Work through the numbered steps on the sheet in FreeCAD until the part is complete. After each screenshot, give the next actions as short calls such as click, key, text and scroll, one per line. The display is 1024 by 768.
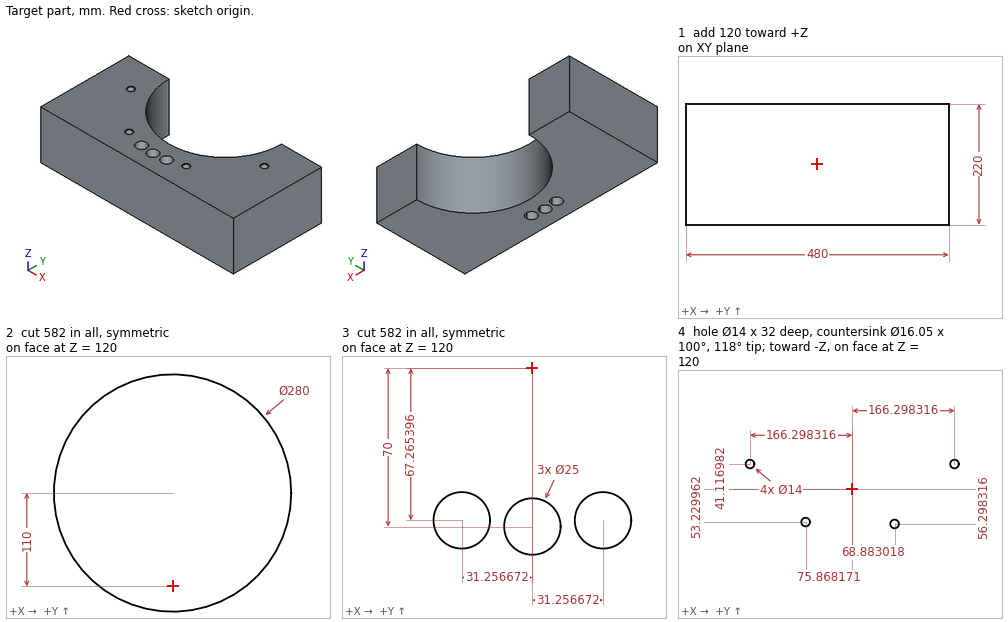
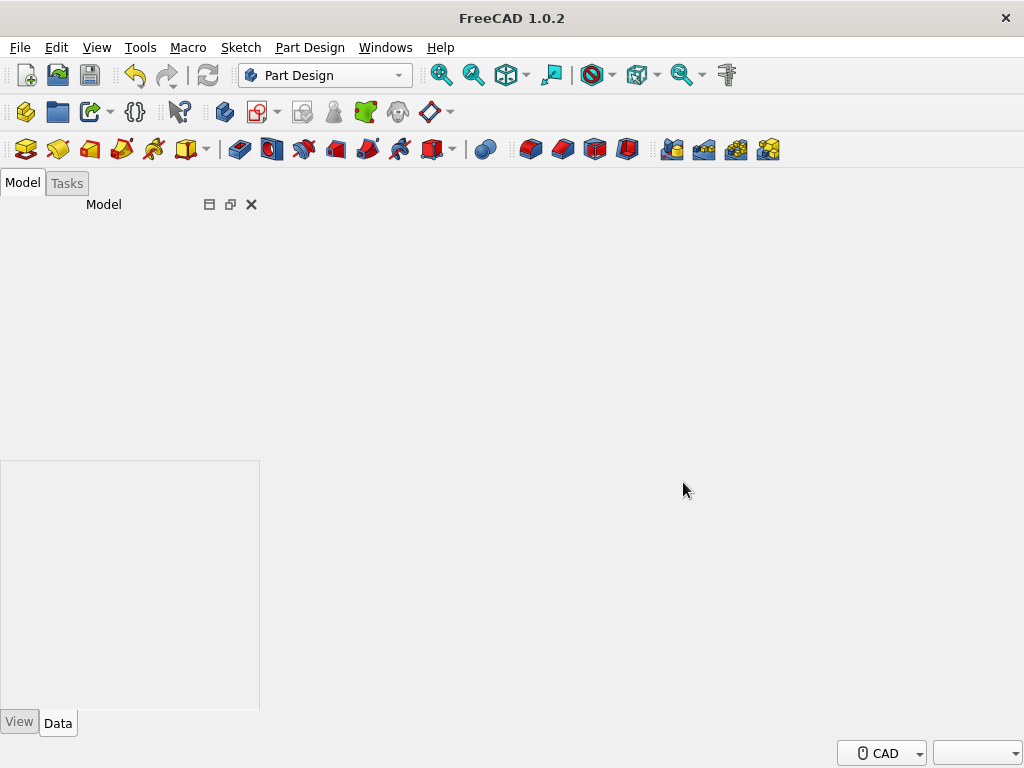
key(ctrl+n)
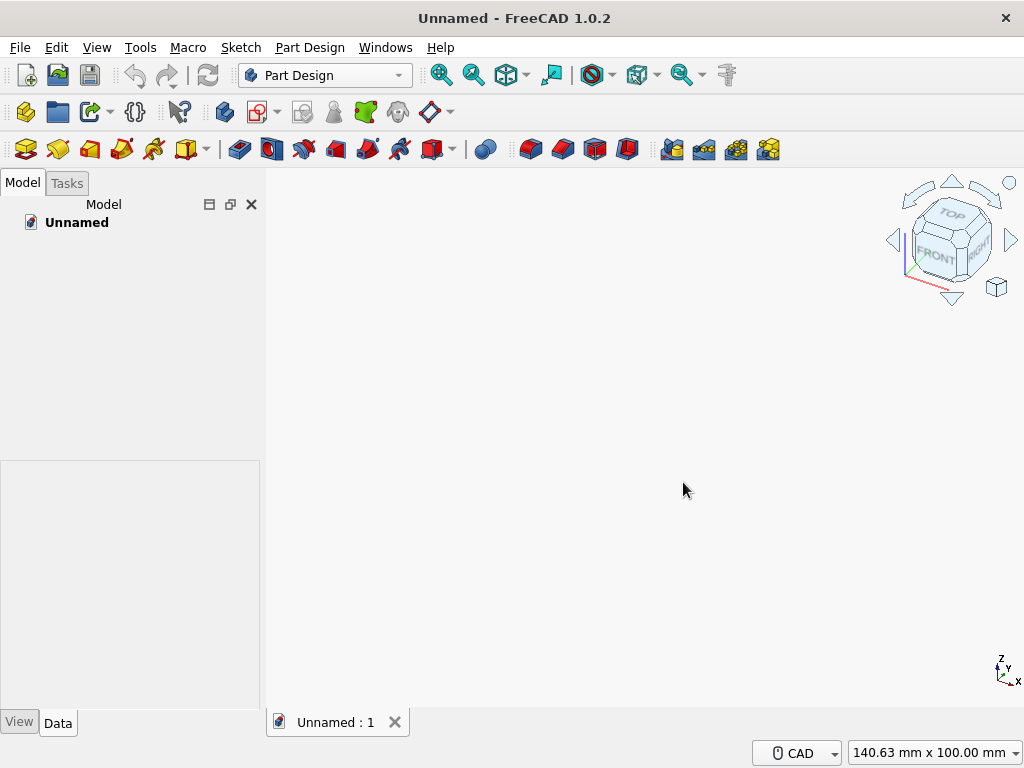
click(258, 112)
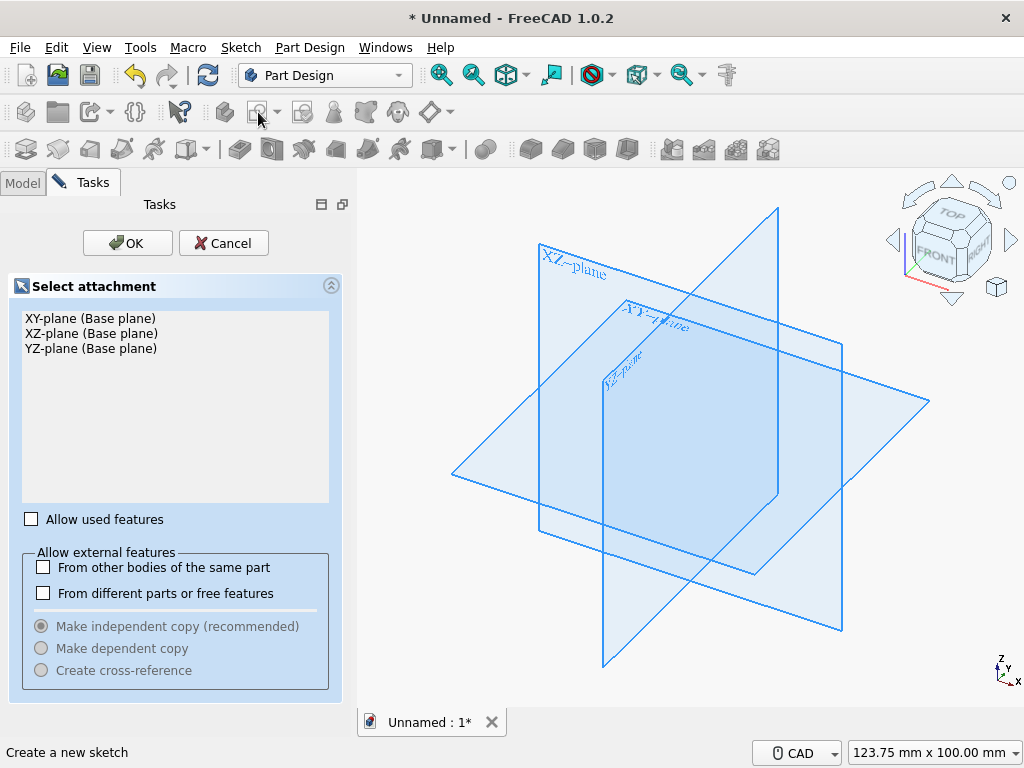
click(82, 318)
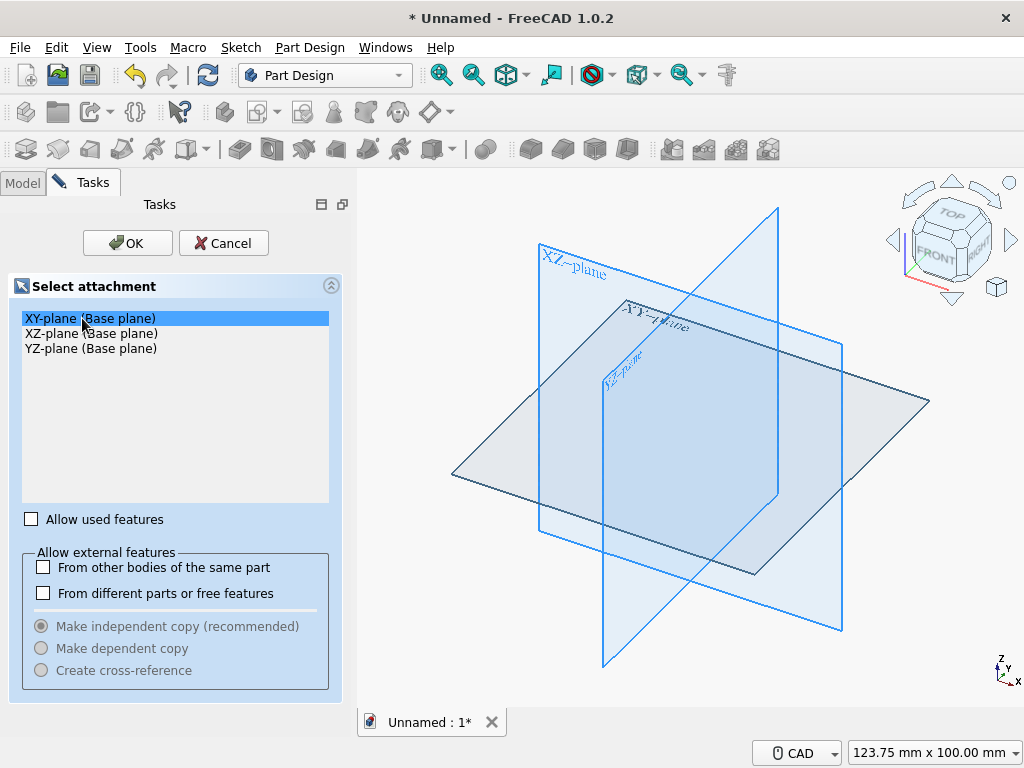
click(128, 243)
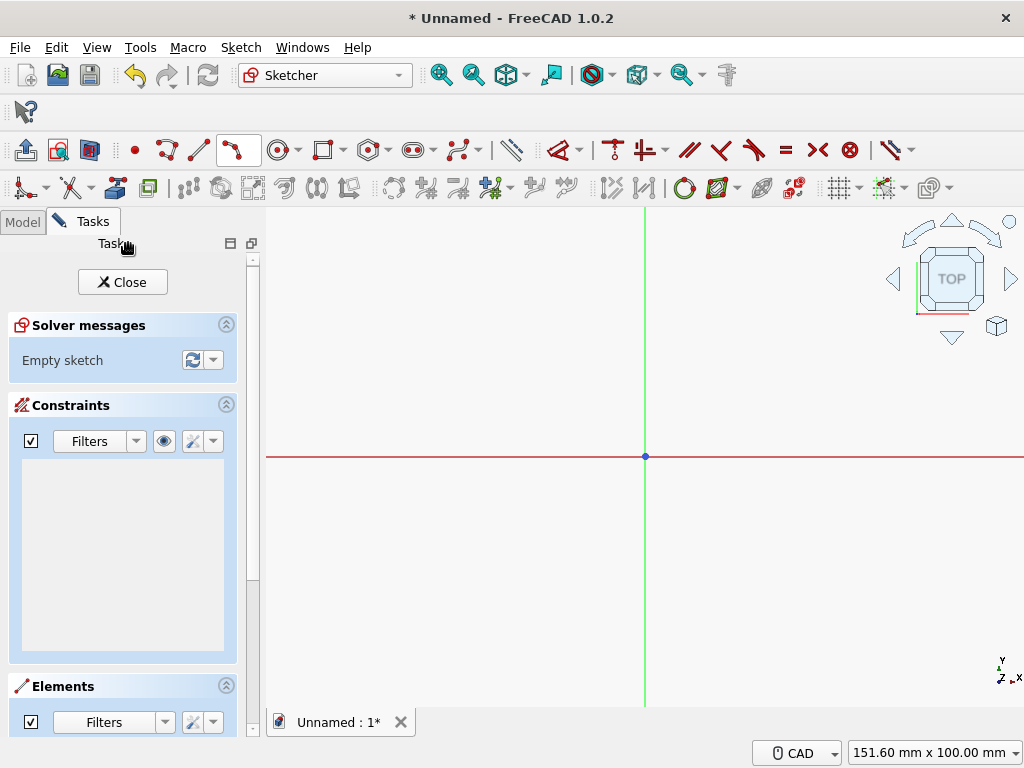
scroll(563, 457, down, 9)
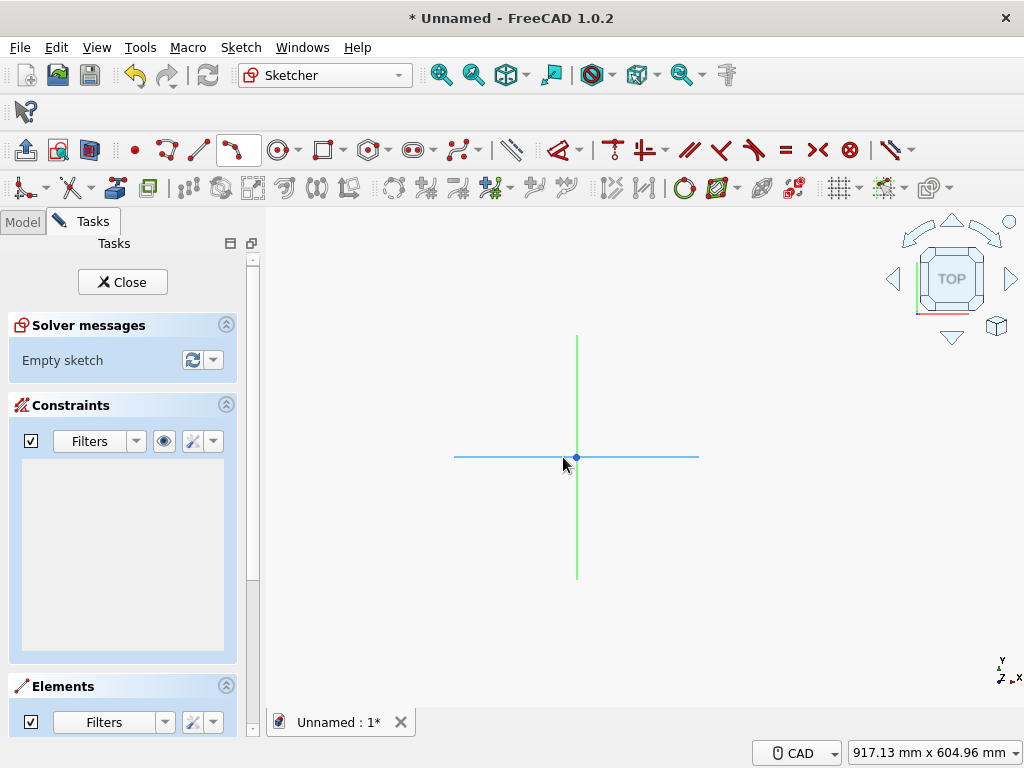
click(346, 150)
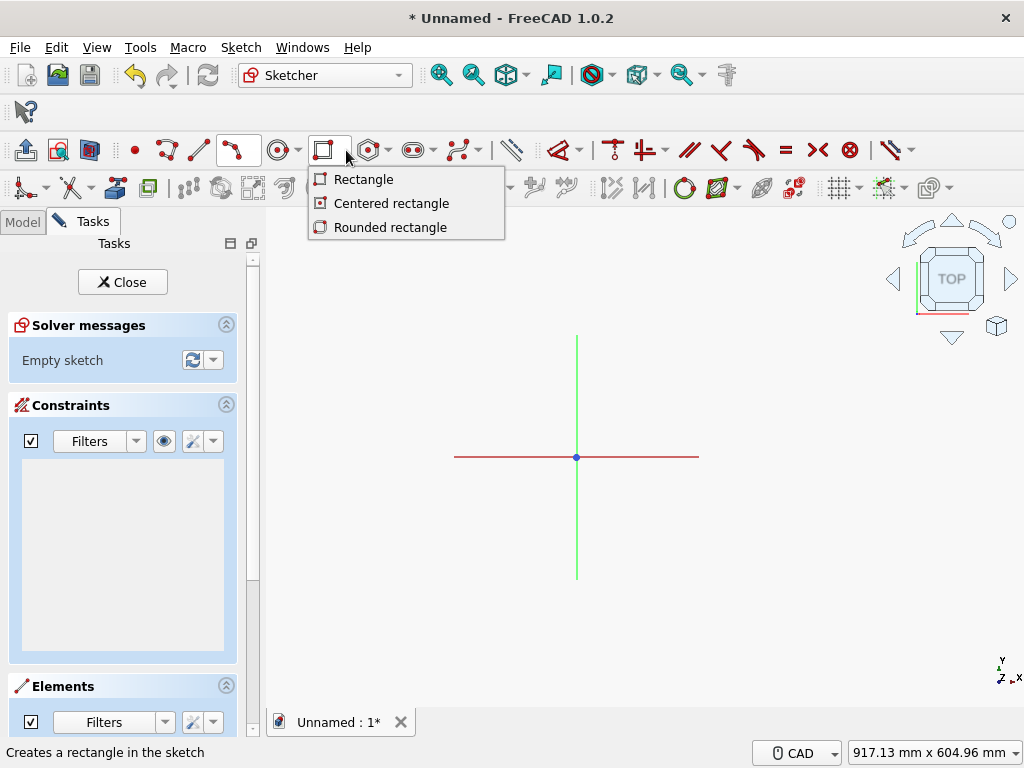
click(406, 203)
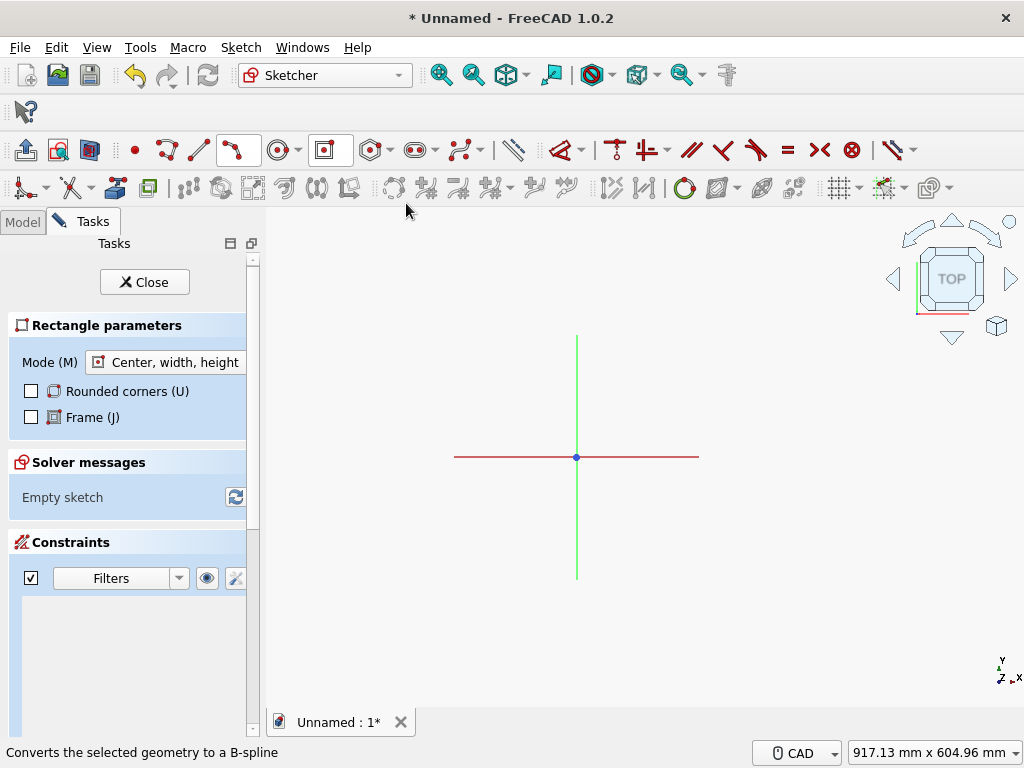
click(577, 457)
move(775, 367)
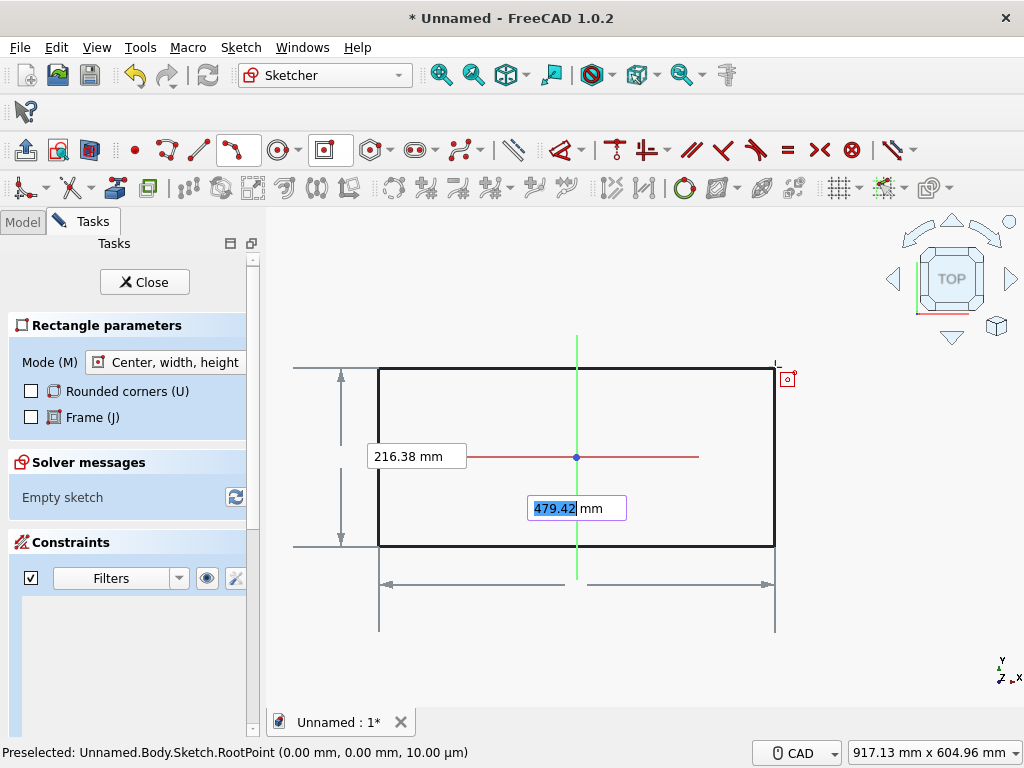
text(480)
key(Tab)
text(220)
key(Return)
key(Escape)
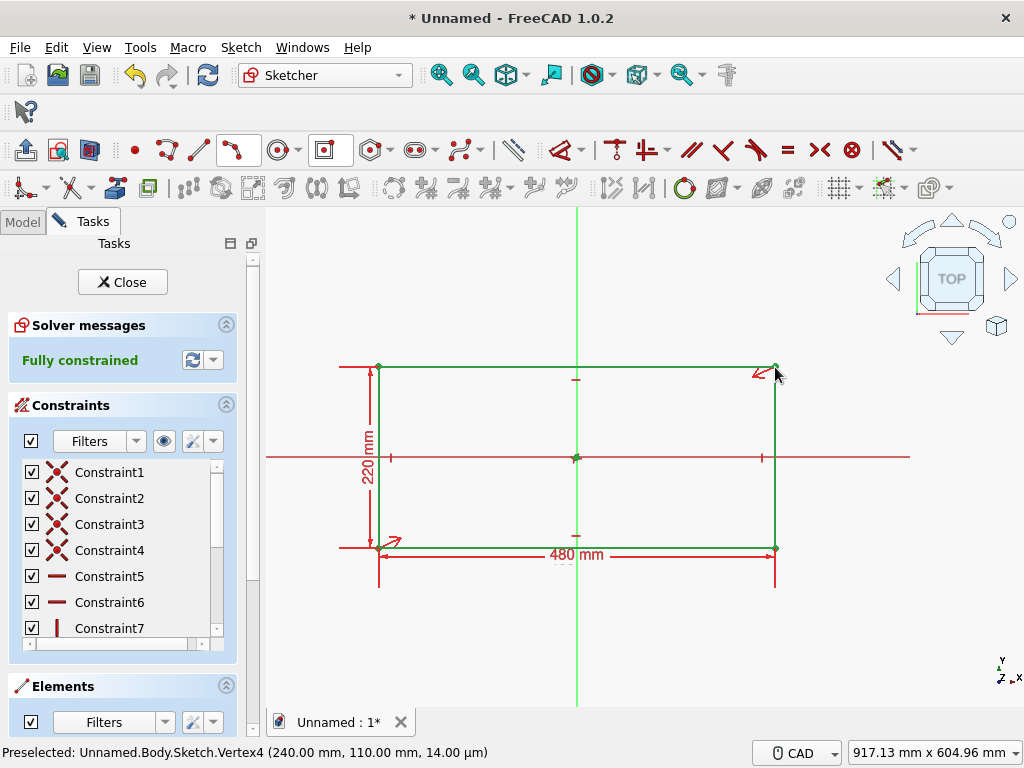
click(123, 282)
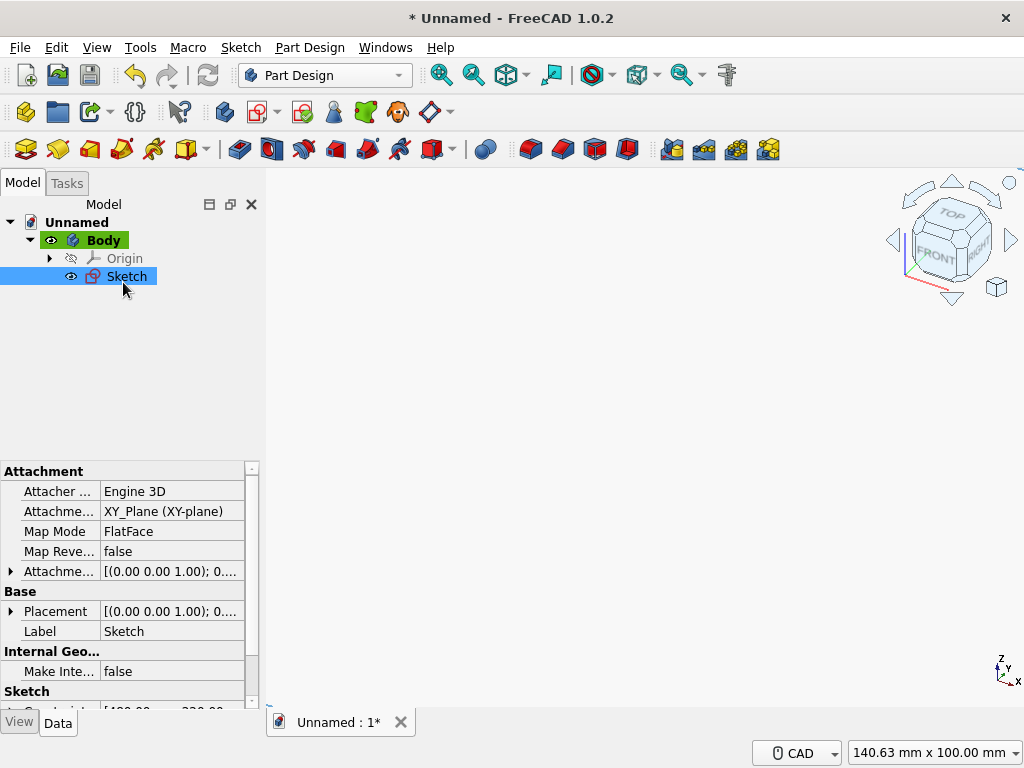
click(26, 150)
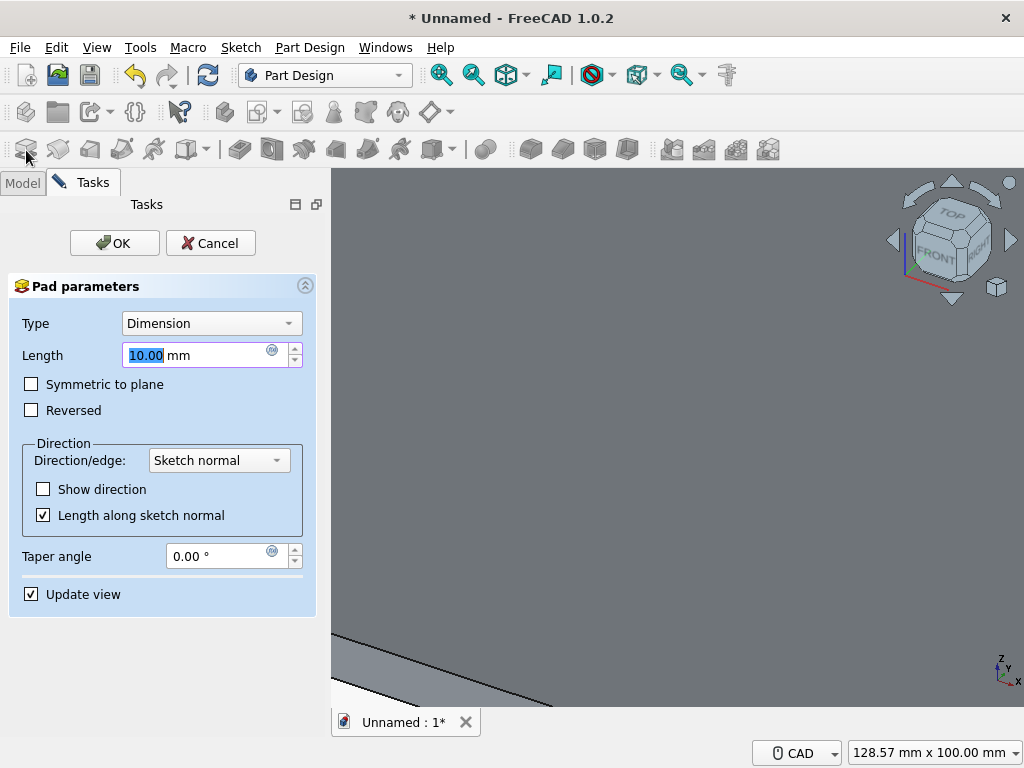
text(120)
key(Tab)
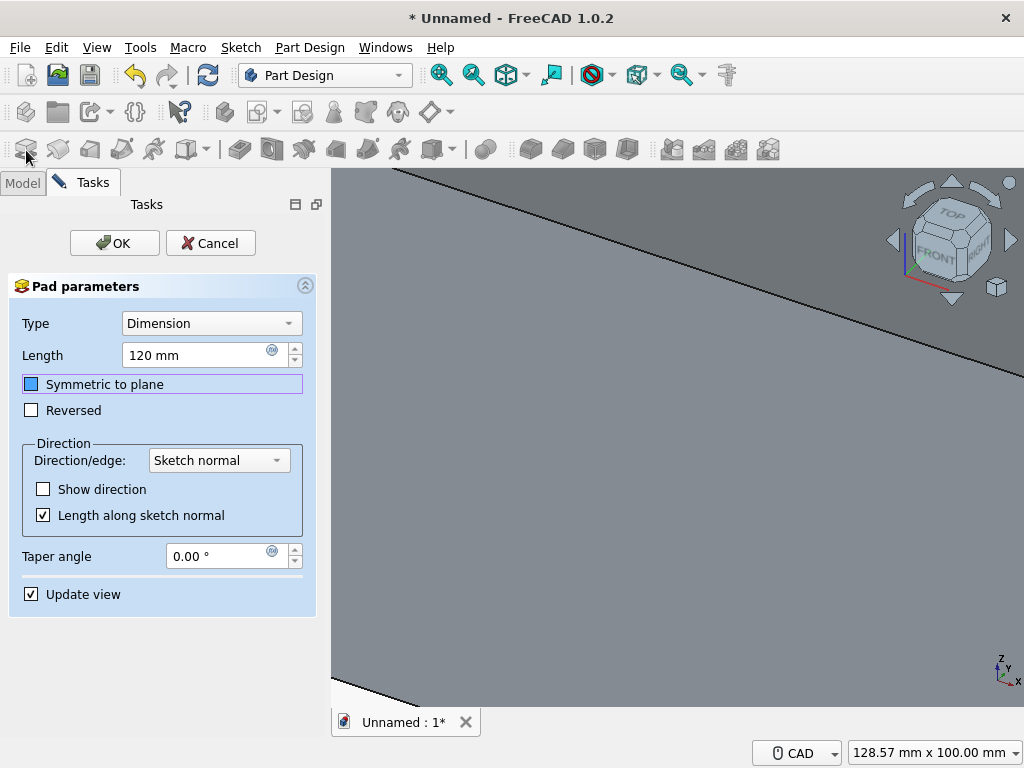
click(115, 243)